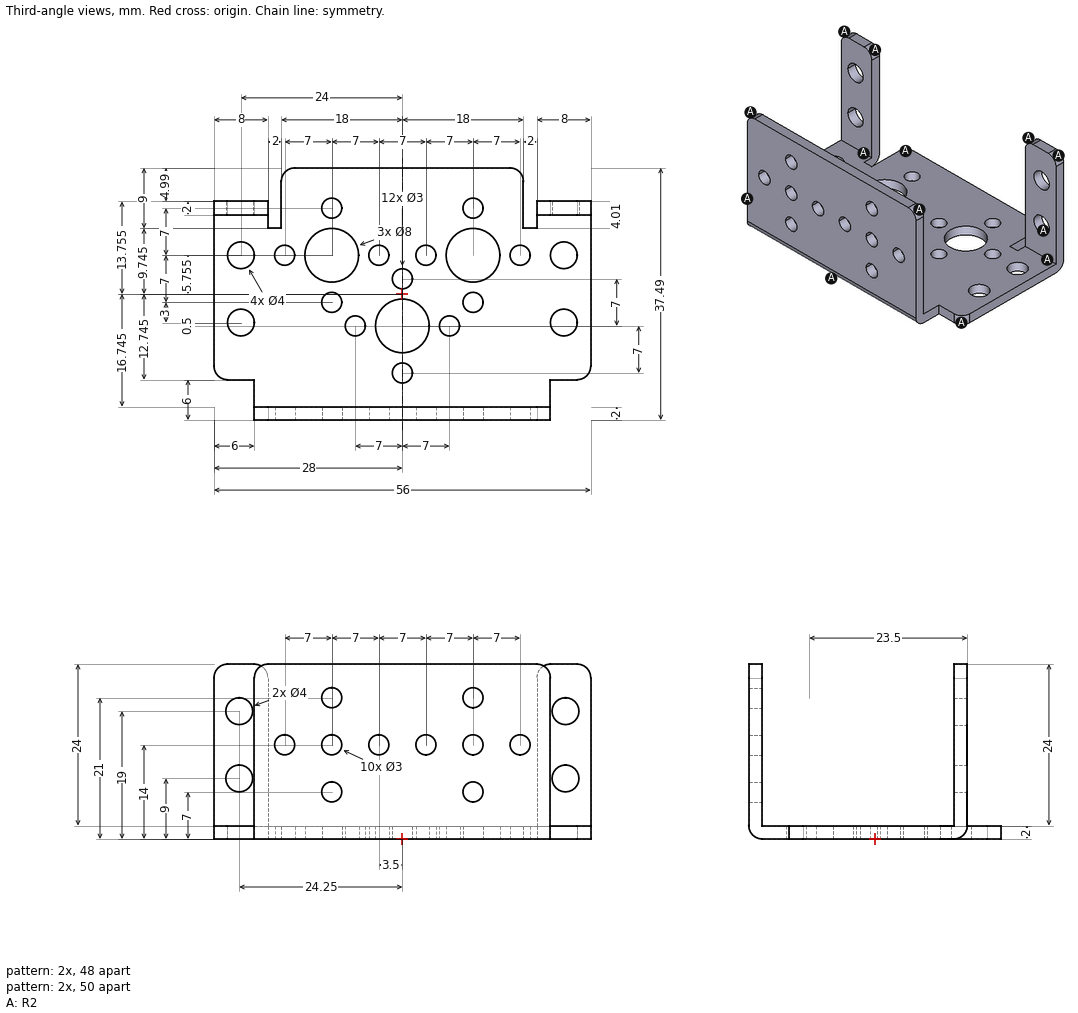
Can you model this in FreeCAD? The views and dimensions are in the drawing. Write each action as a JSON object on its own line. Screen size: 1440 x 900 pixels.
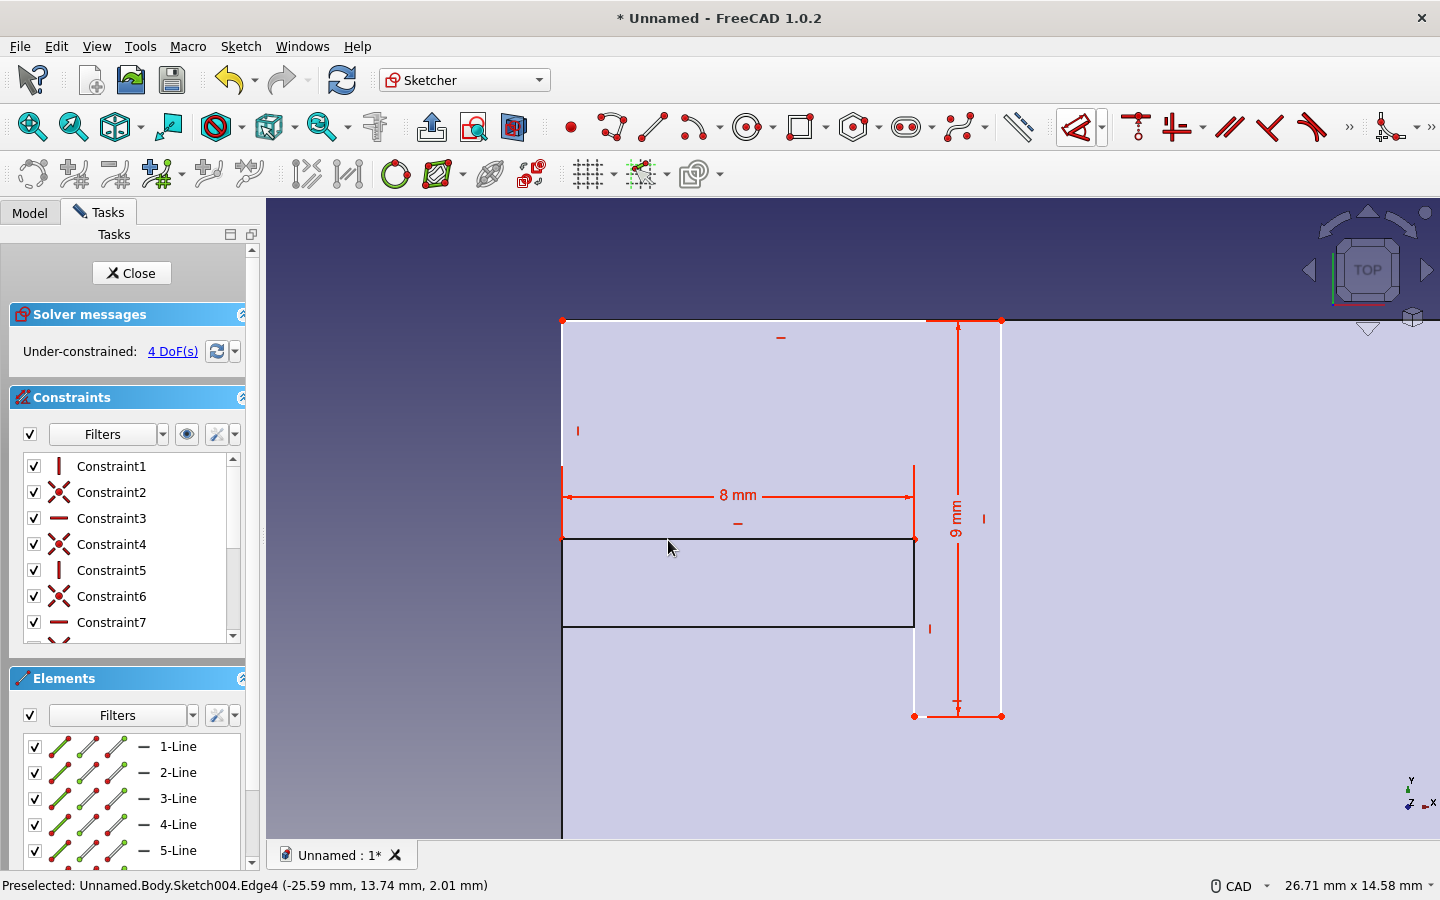
{"action": "left_click", "coordinate": [940, 717]}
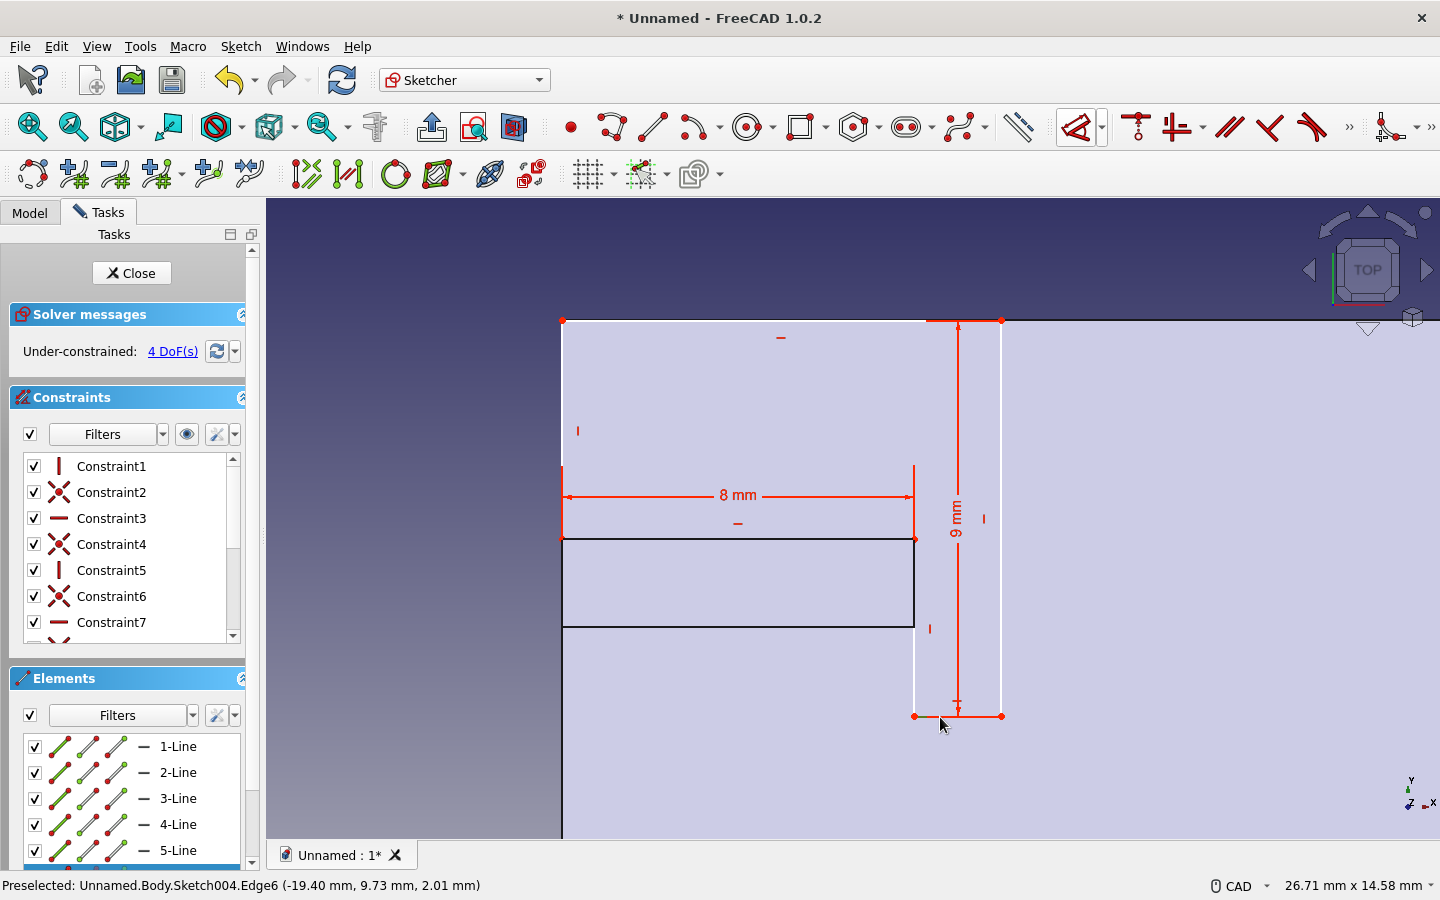
{"action": "key", "text": "l"}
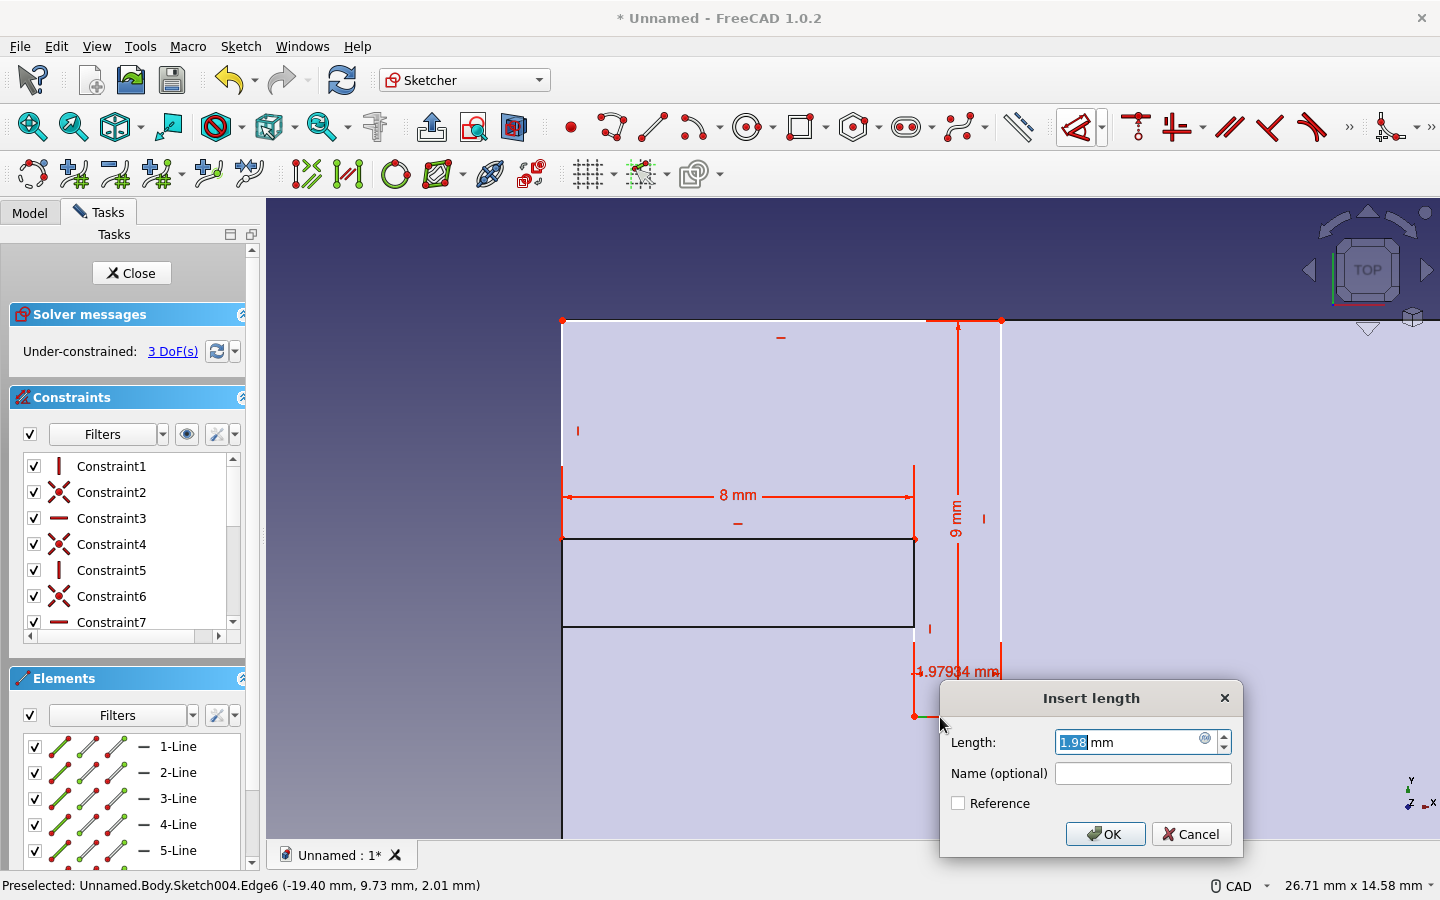
{"action": "type", "text": "2"}
{"action": "key", "text": "Return"}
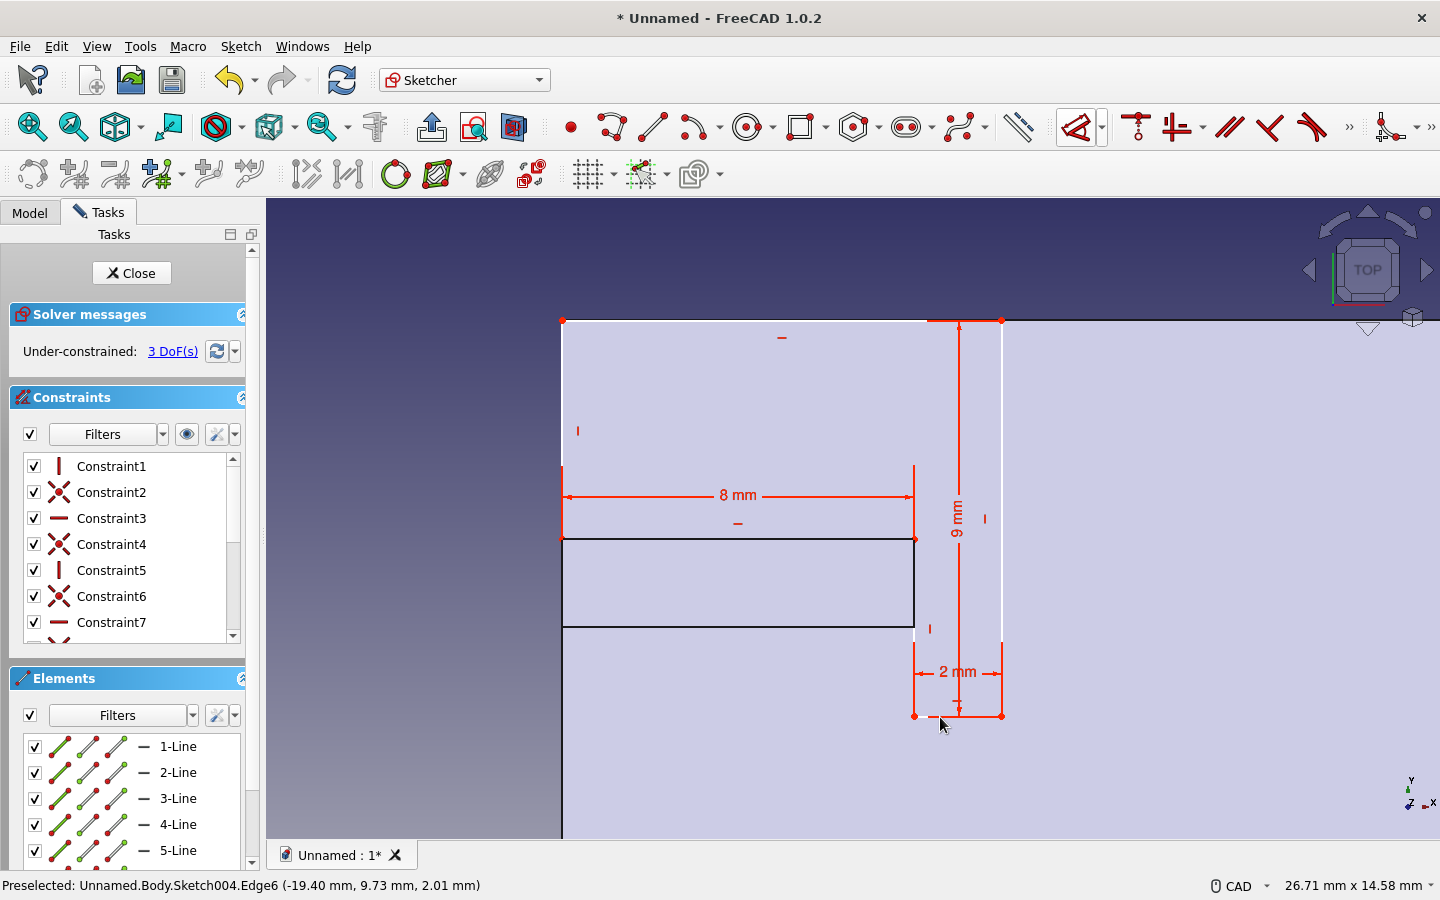
{"action": "left_click", "coordinate": [1002, 717]}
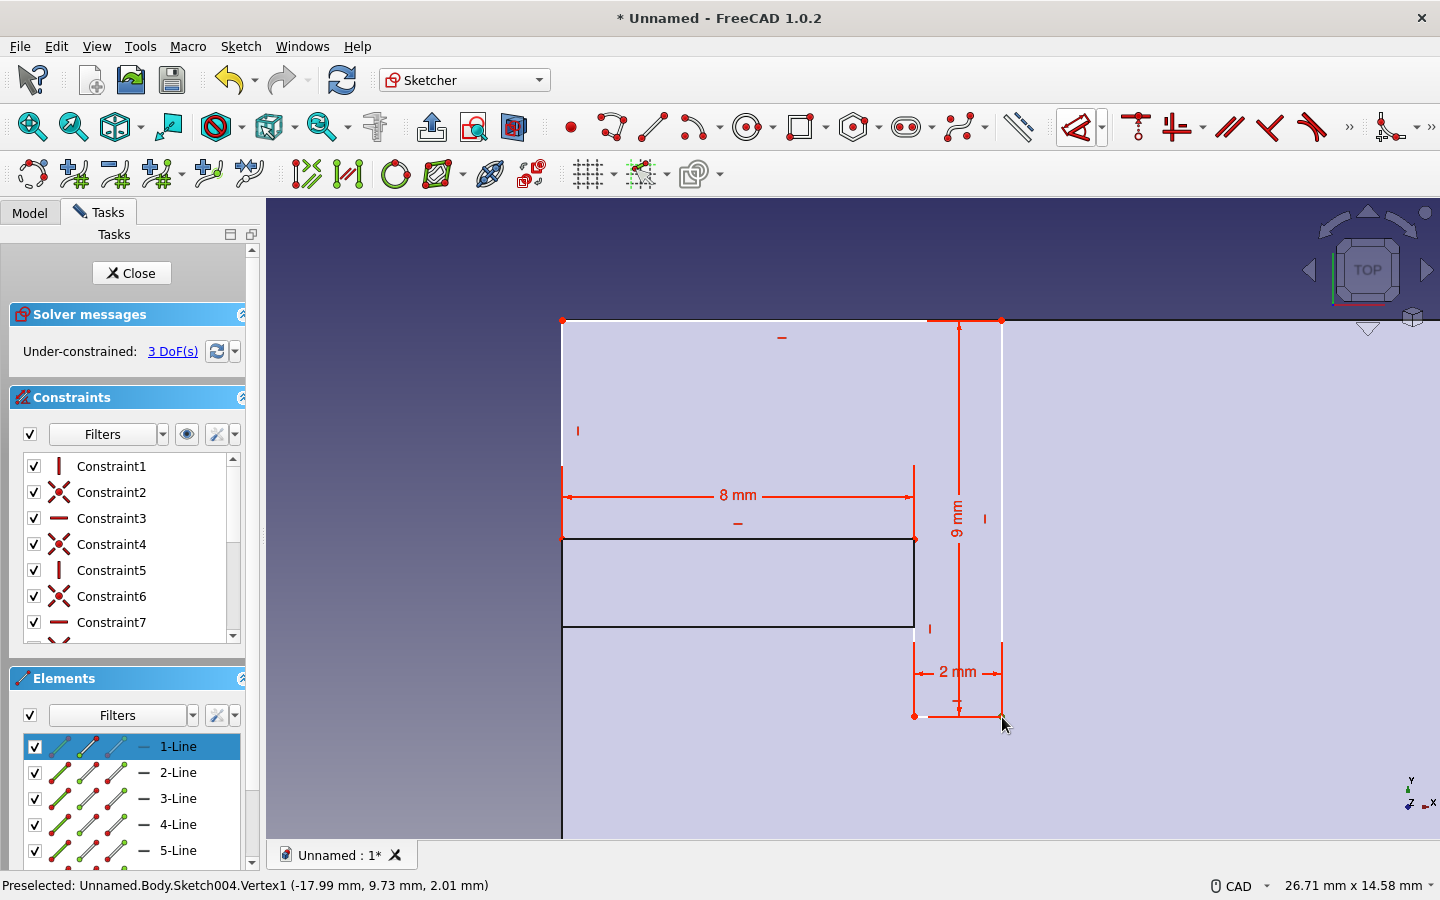
{"action": "key", "text": "l"}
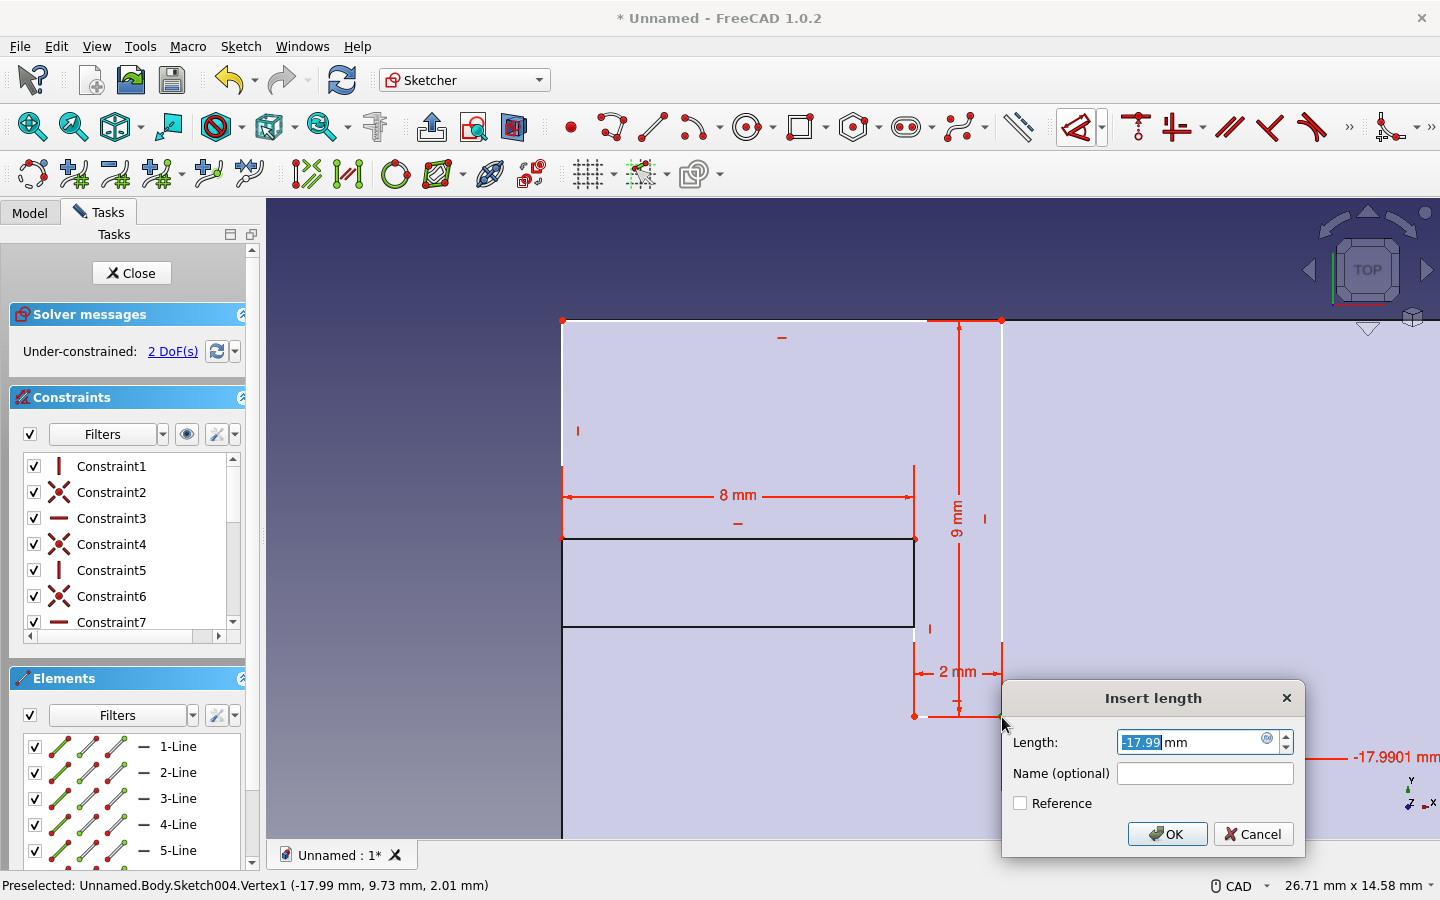
{"action": "type", "text": "-18"}
{"action": "key", "text": "Return"}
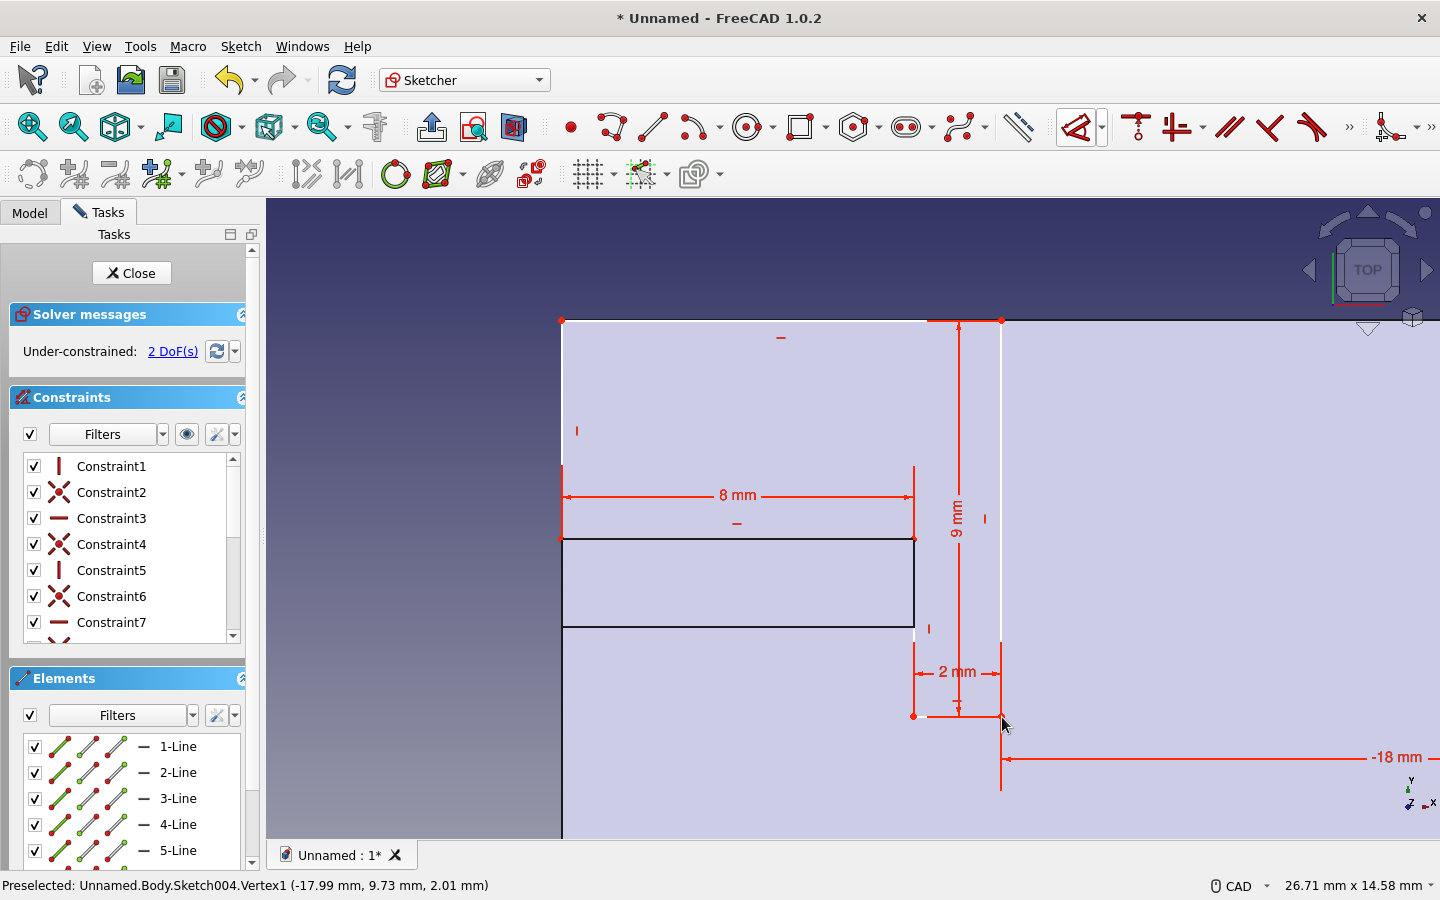
{"action": "left_click", "coordinate": [562, 387]}